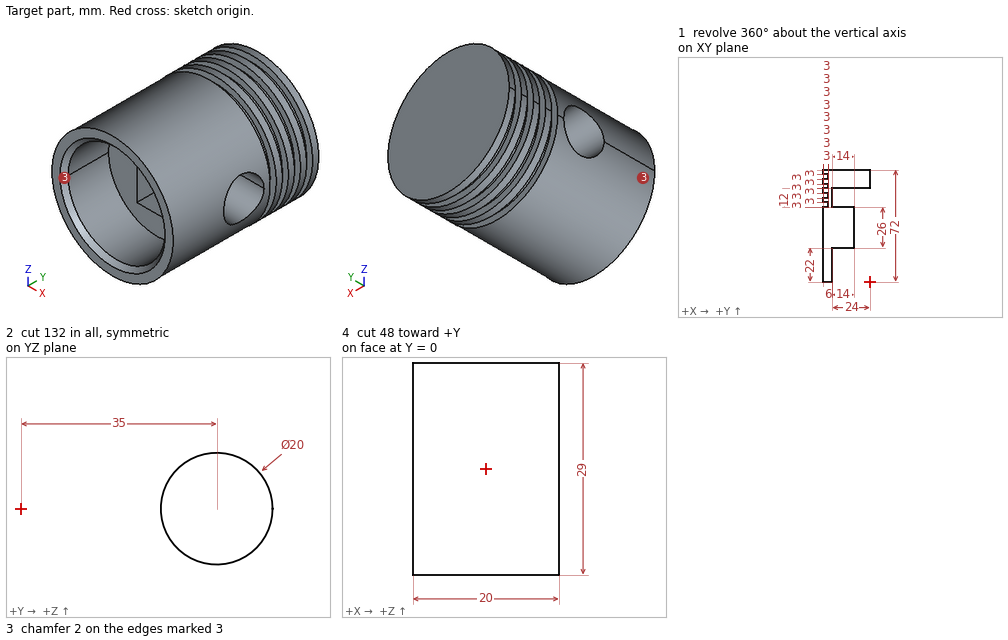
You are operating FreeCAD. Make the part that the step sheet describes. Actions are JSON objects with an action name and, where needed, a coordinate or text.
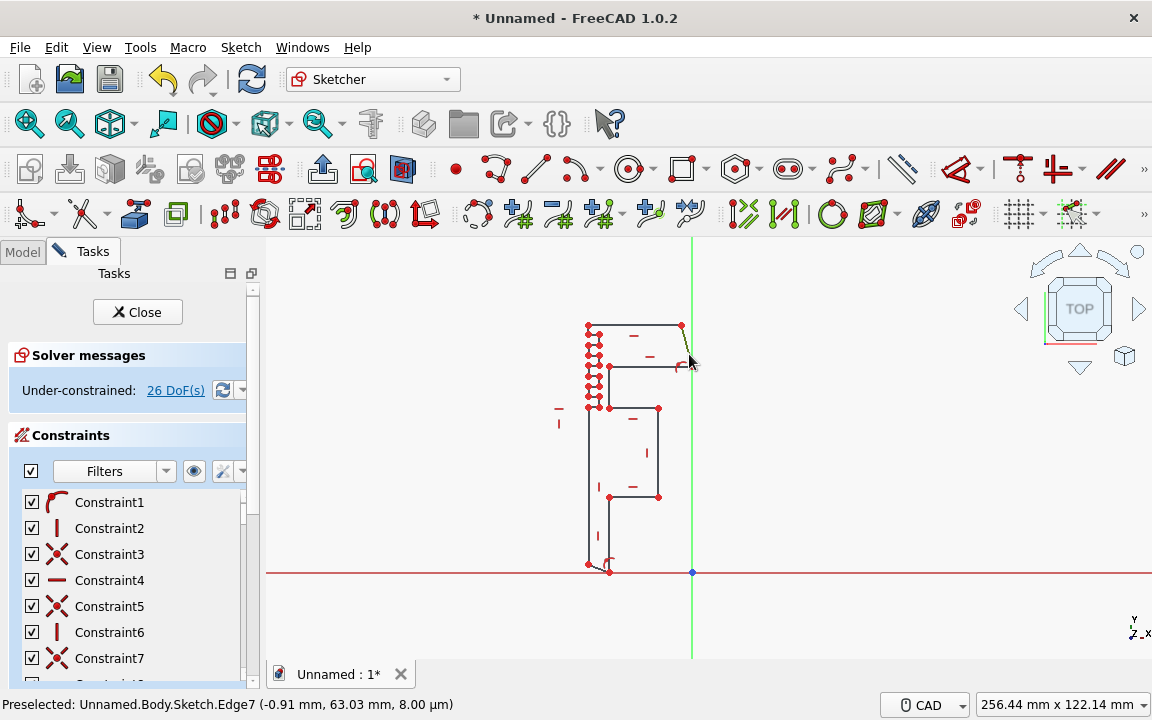
{"action": "key", "text": "v"}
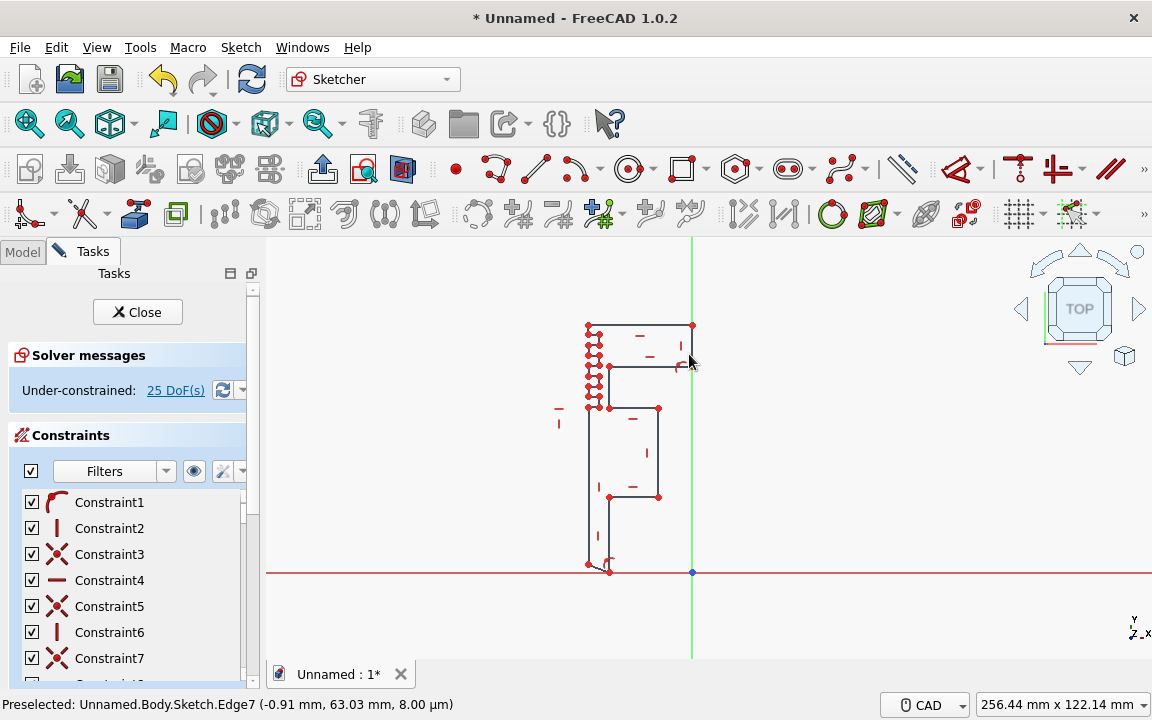
{"action": "scroll", "coordinate": [599, 569], "scroll_direction": "up", "scroll_amount": 2}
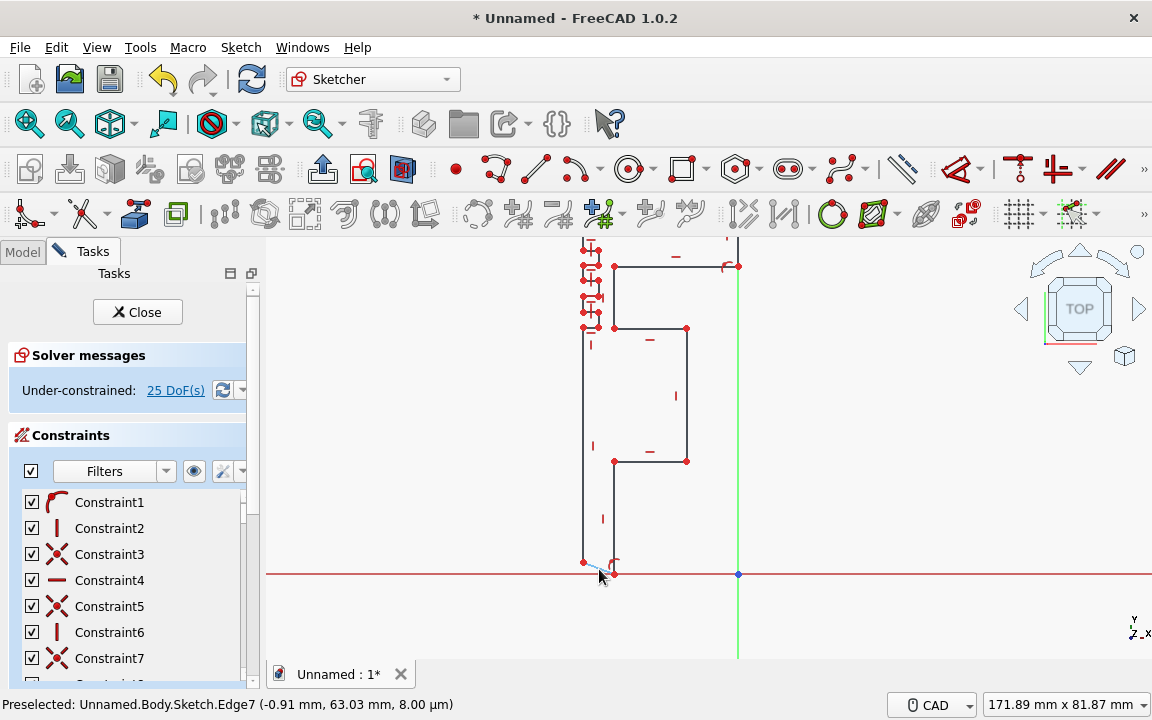
{"action": "left_click", "coordinate": [599, 568]}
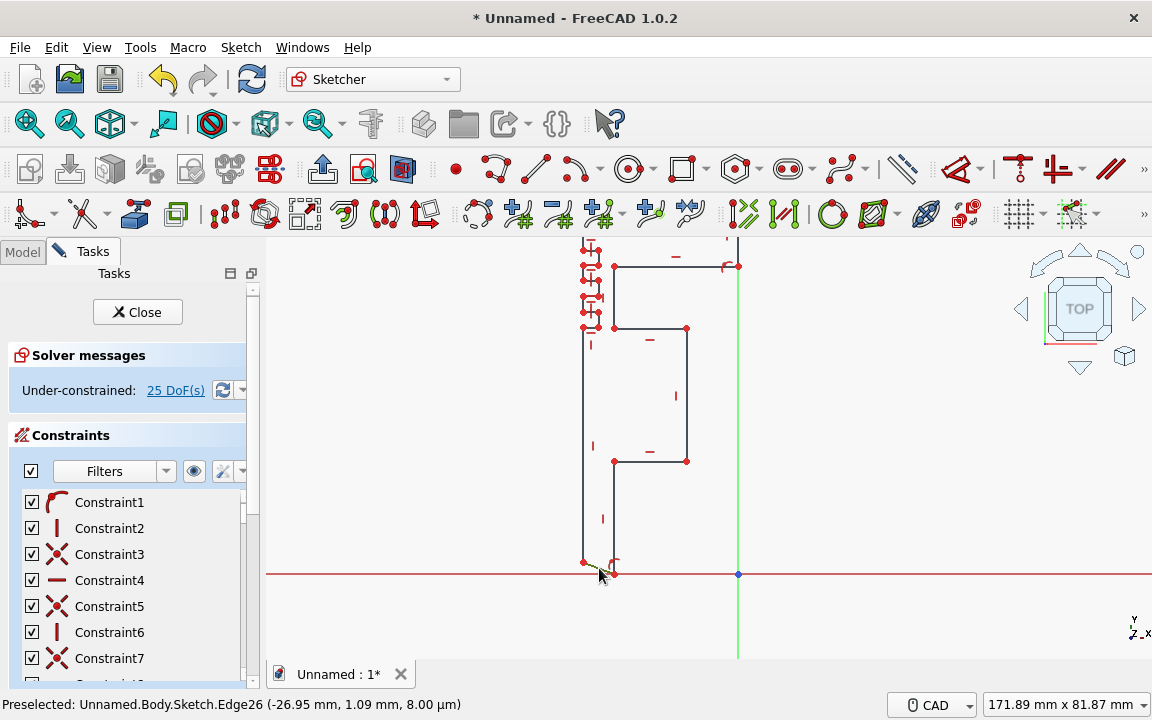
{"action": "key", "text": "h"}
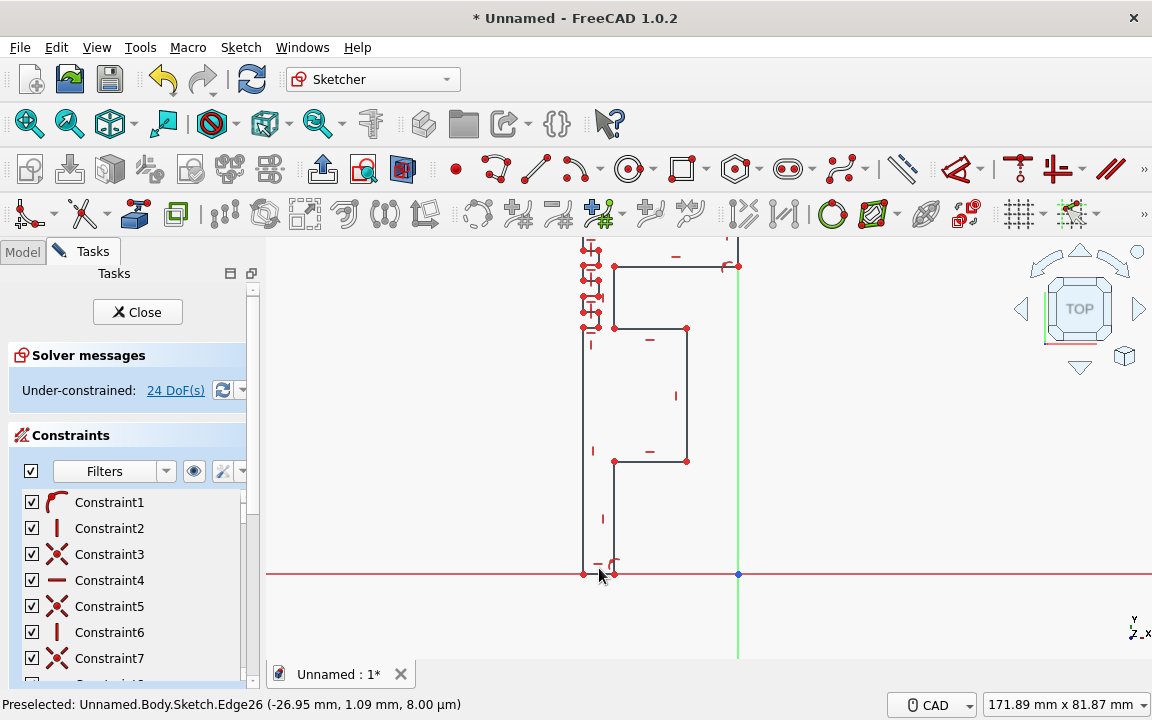
{"action": "scroll", "coordinate": [599, 569], "scroll_direction": "down", "scroll_amount": 2}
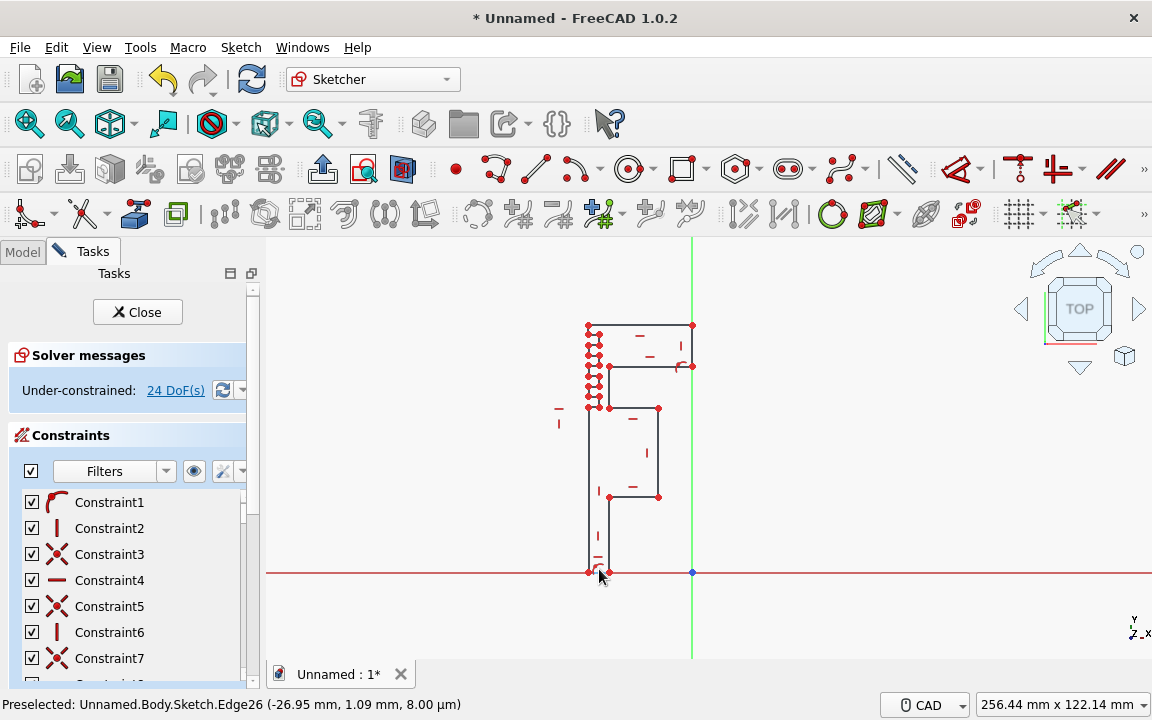
{"action": "scroll", "coordinate": [588, 330], "scroll_direction": "up", "scroll_amount": 7}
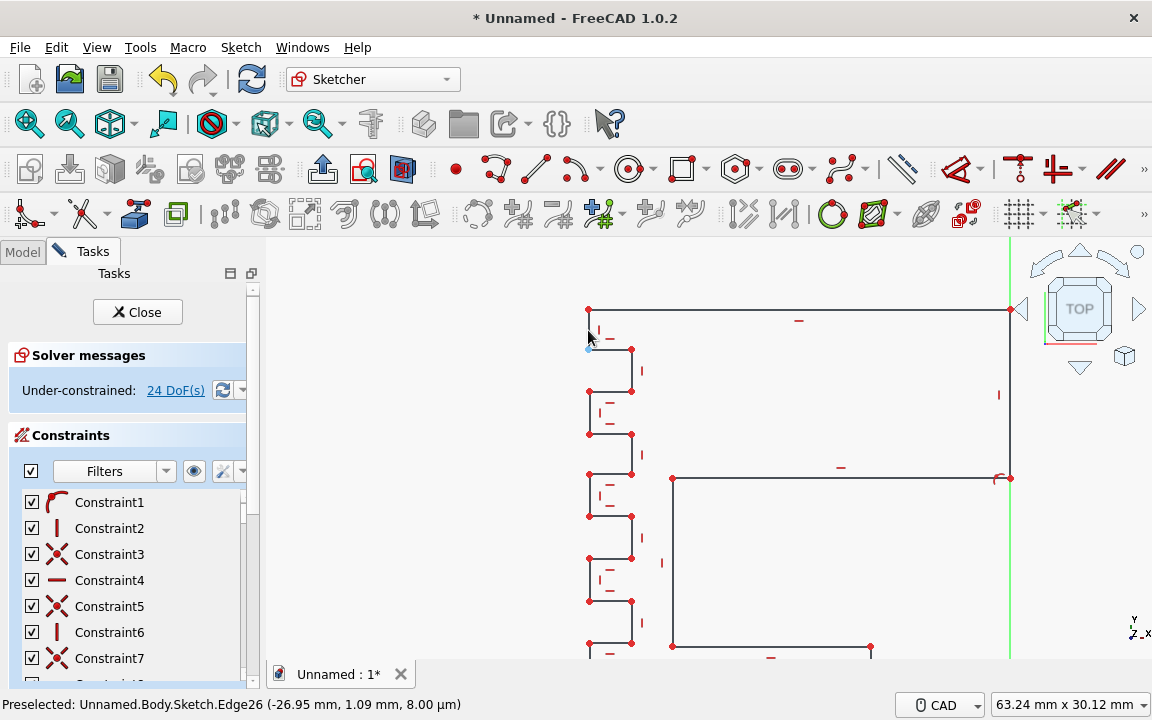
{"action": "left_click", "coordinate": [589, 330]}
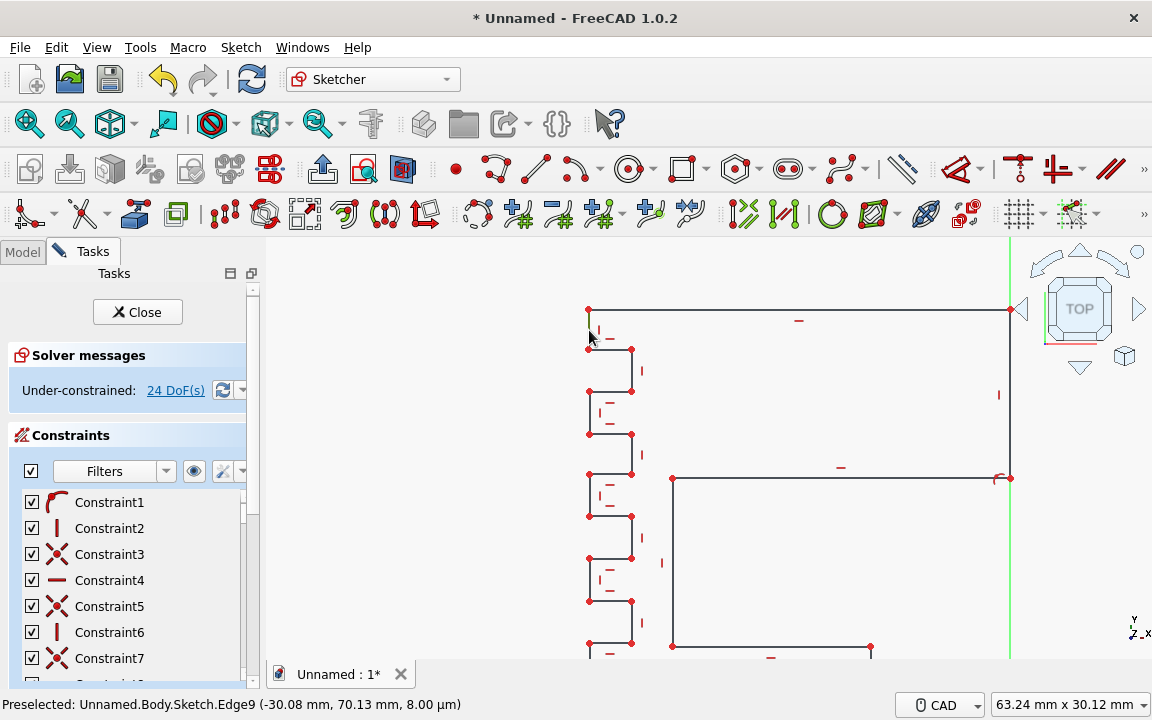
{"action": "left_click", "coordinate": [982, 170]}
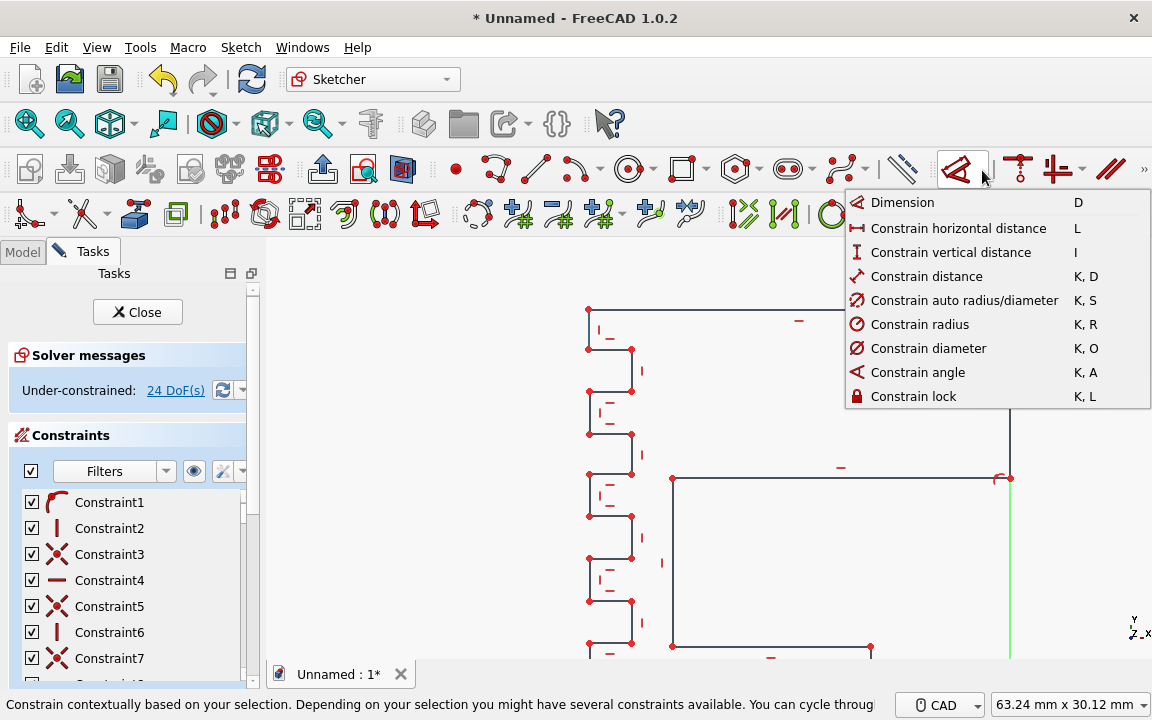
{"action": "left_click", "coordinate": [998, 252]}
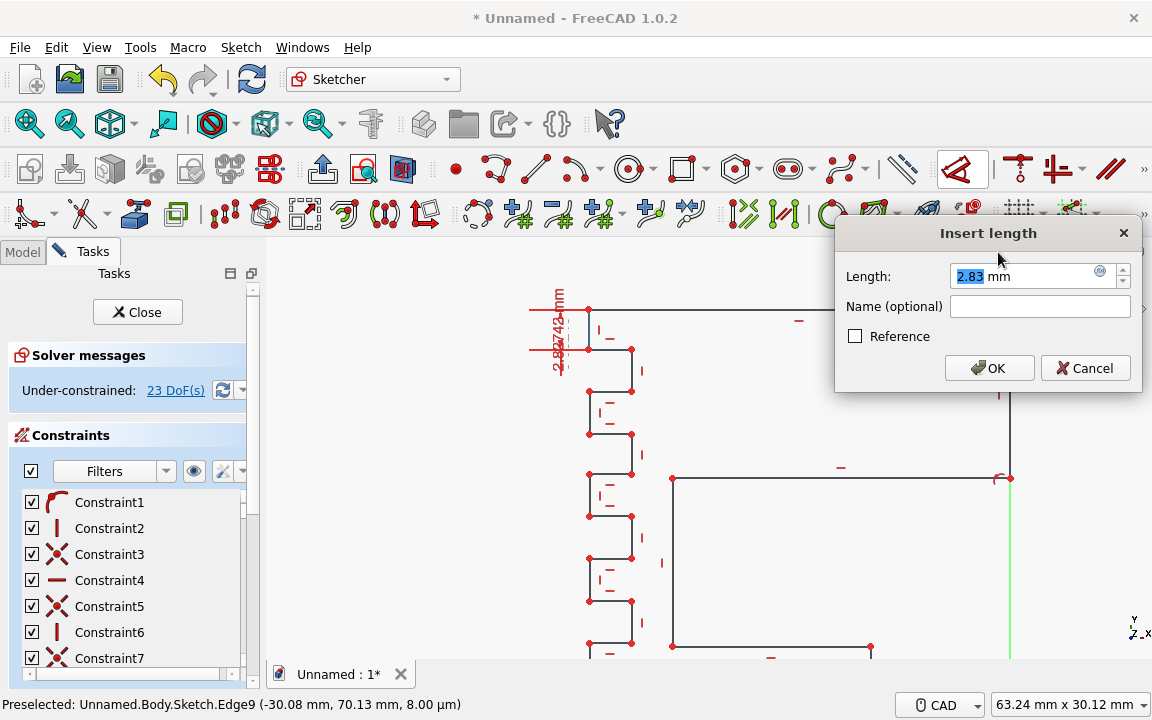
{"action": "type", "text": "3"}
{"action": "key", "text": "Return"}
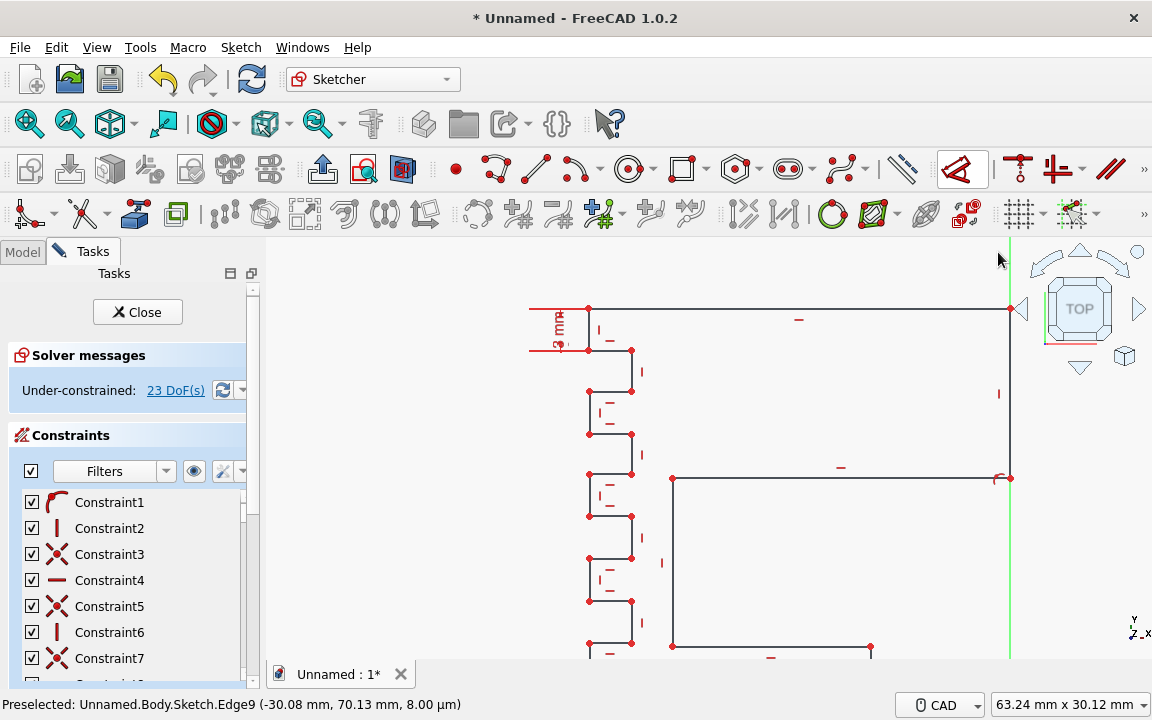
{"action": "left_click", "coordinate": [602, 351]}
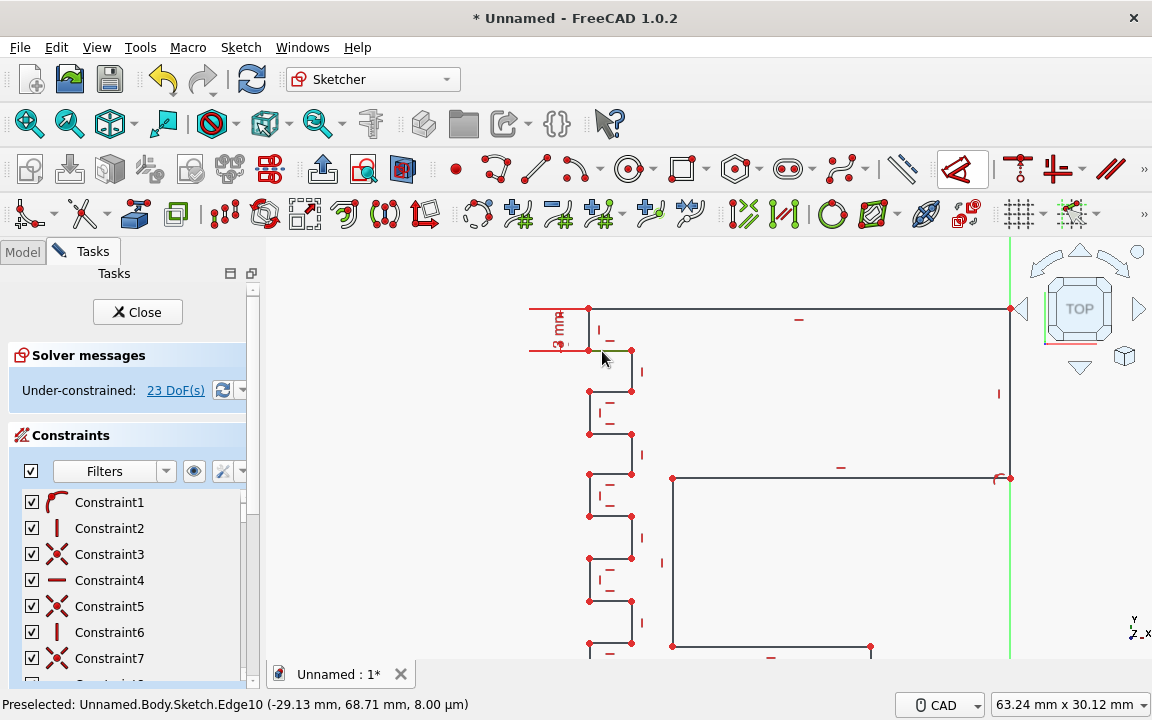
{"action": "key", "text": "l"}